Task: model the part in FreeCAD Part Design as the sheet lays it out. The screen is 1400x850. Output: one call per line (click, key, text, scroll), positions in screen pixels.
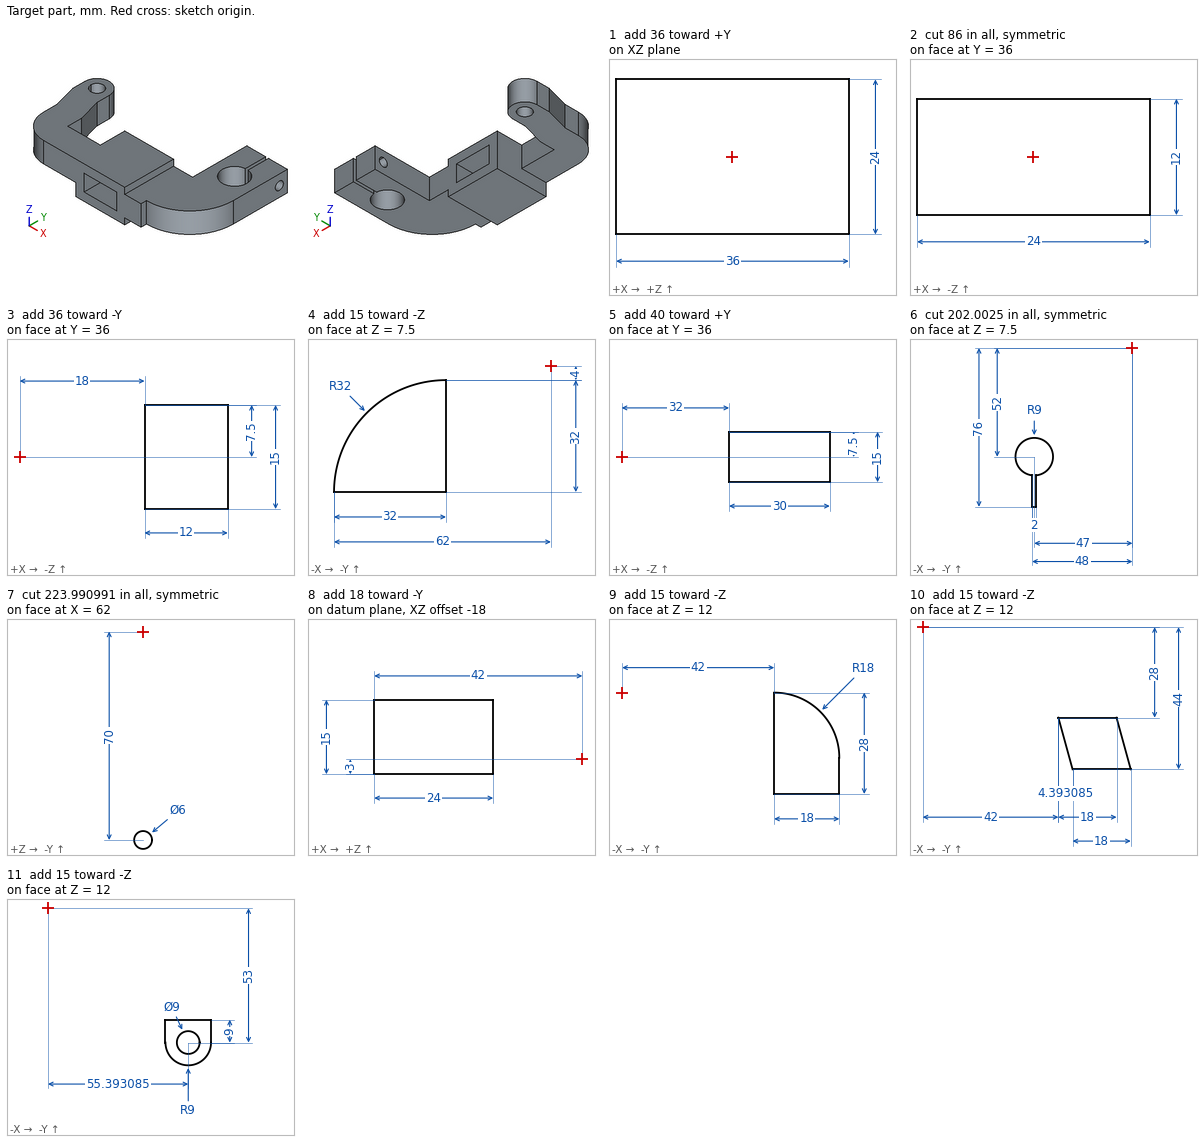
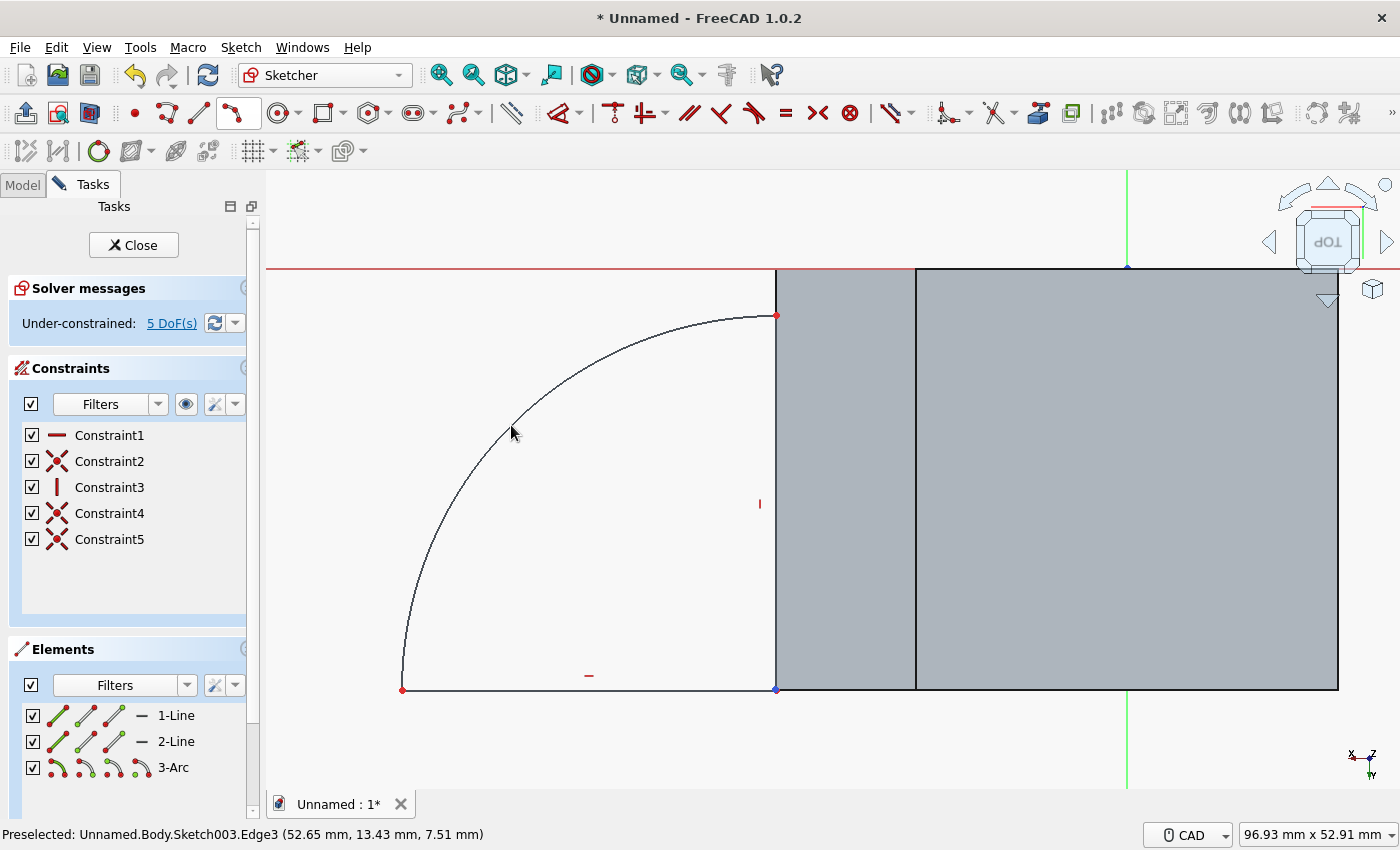
key(d)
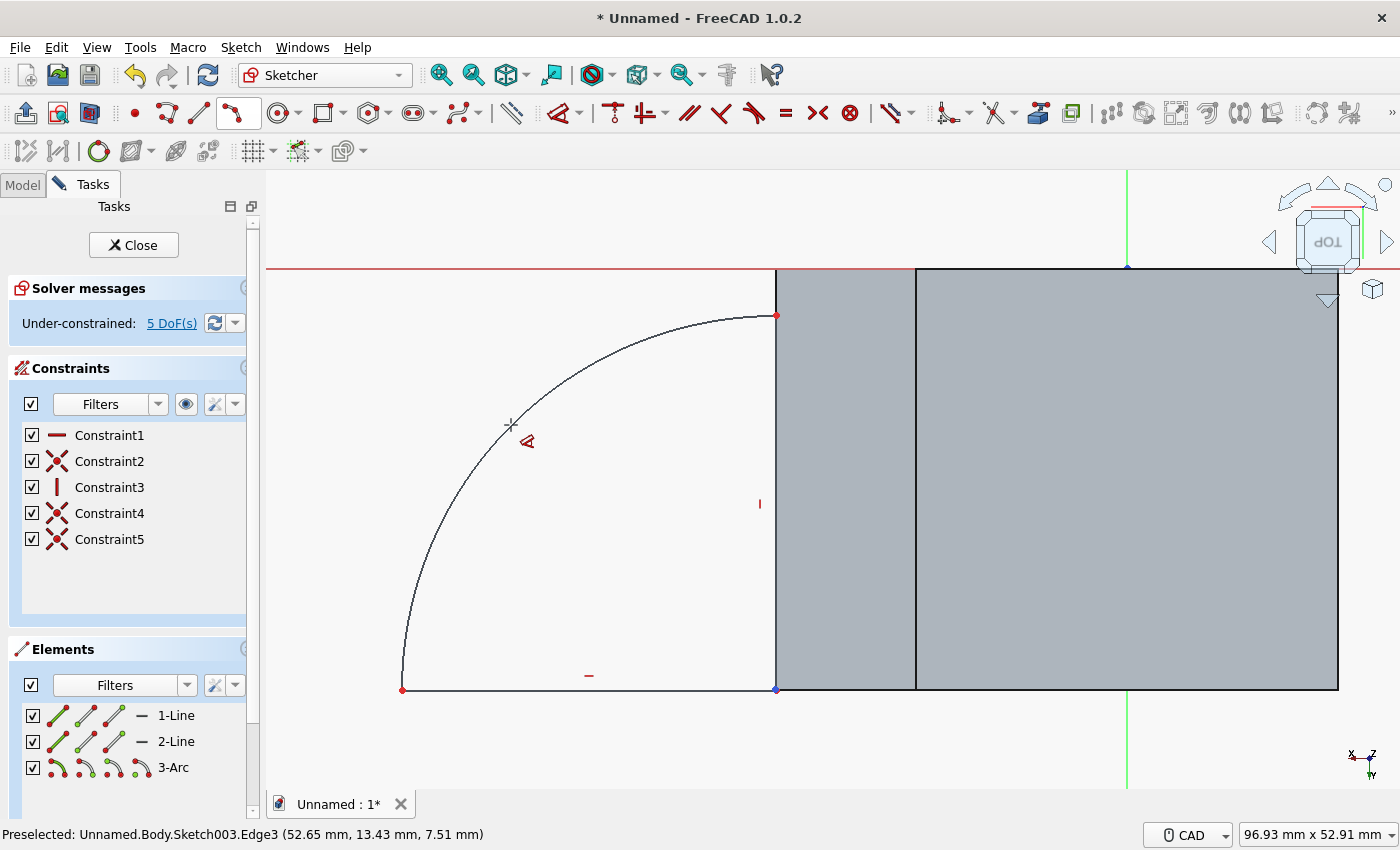
click(606, 357)
click(591, 328)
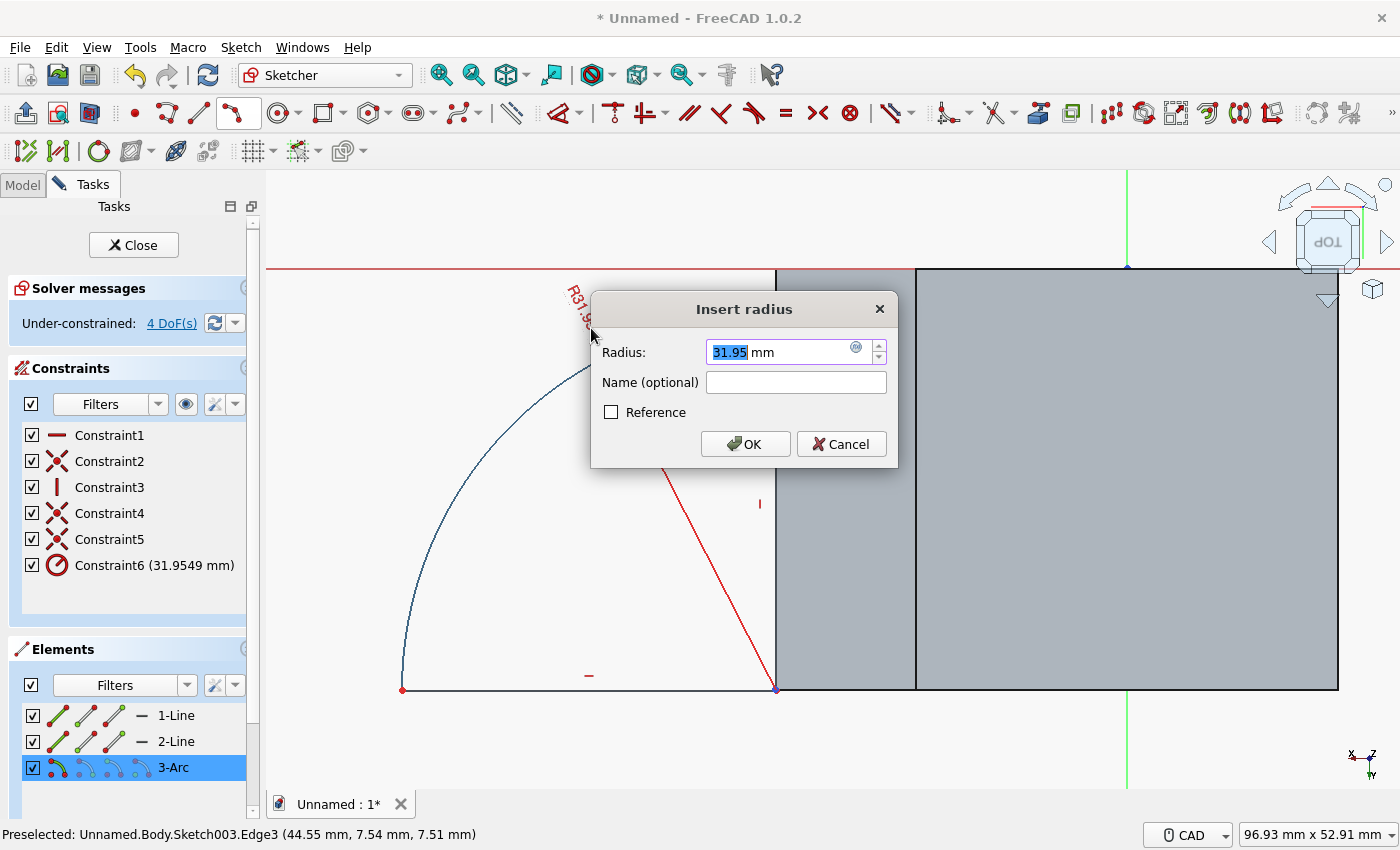
text(32)
key(Return)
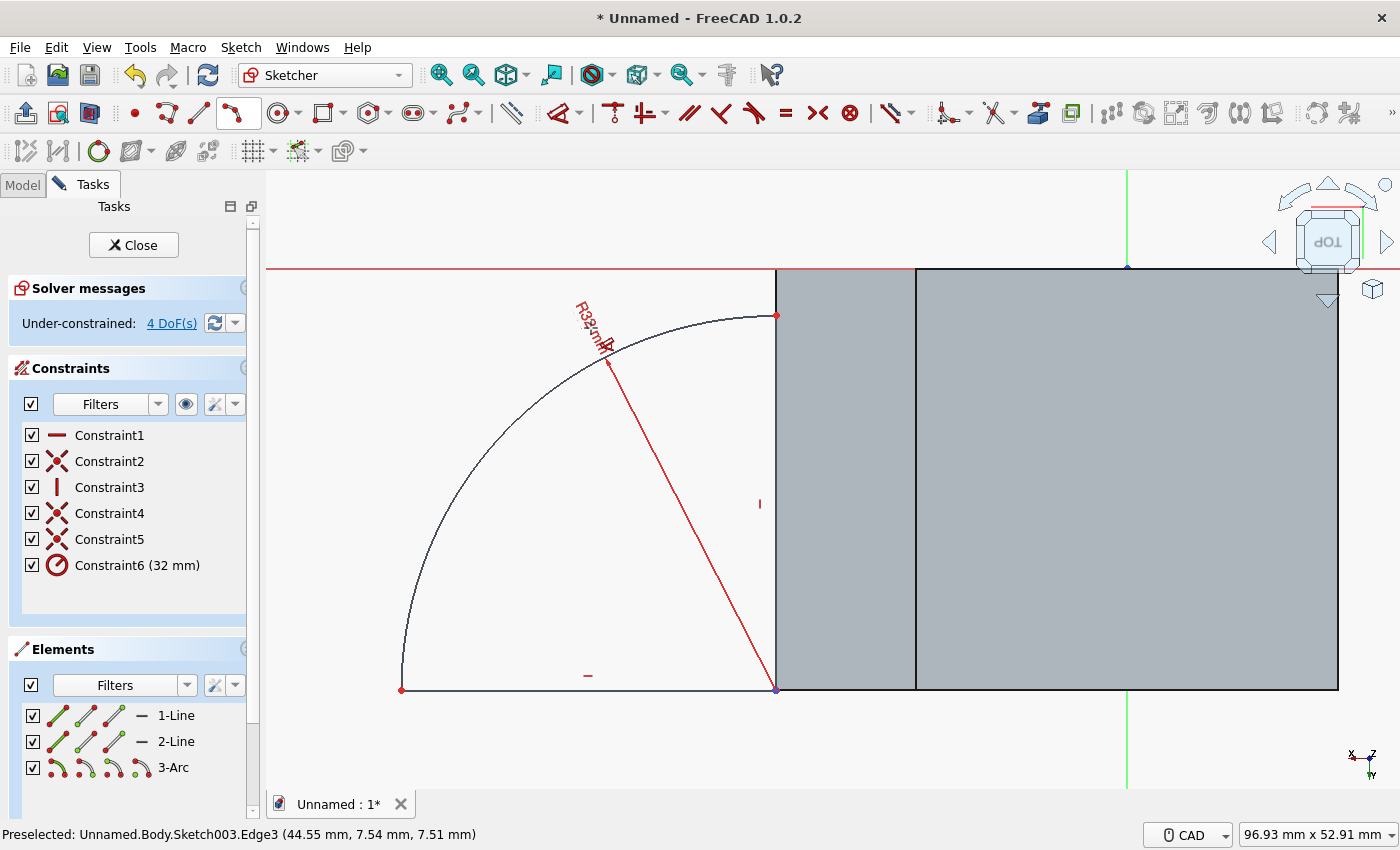
click(514, 691)
click(589, 725)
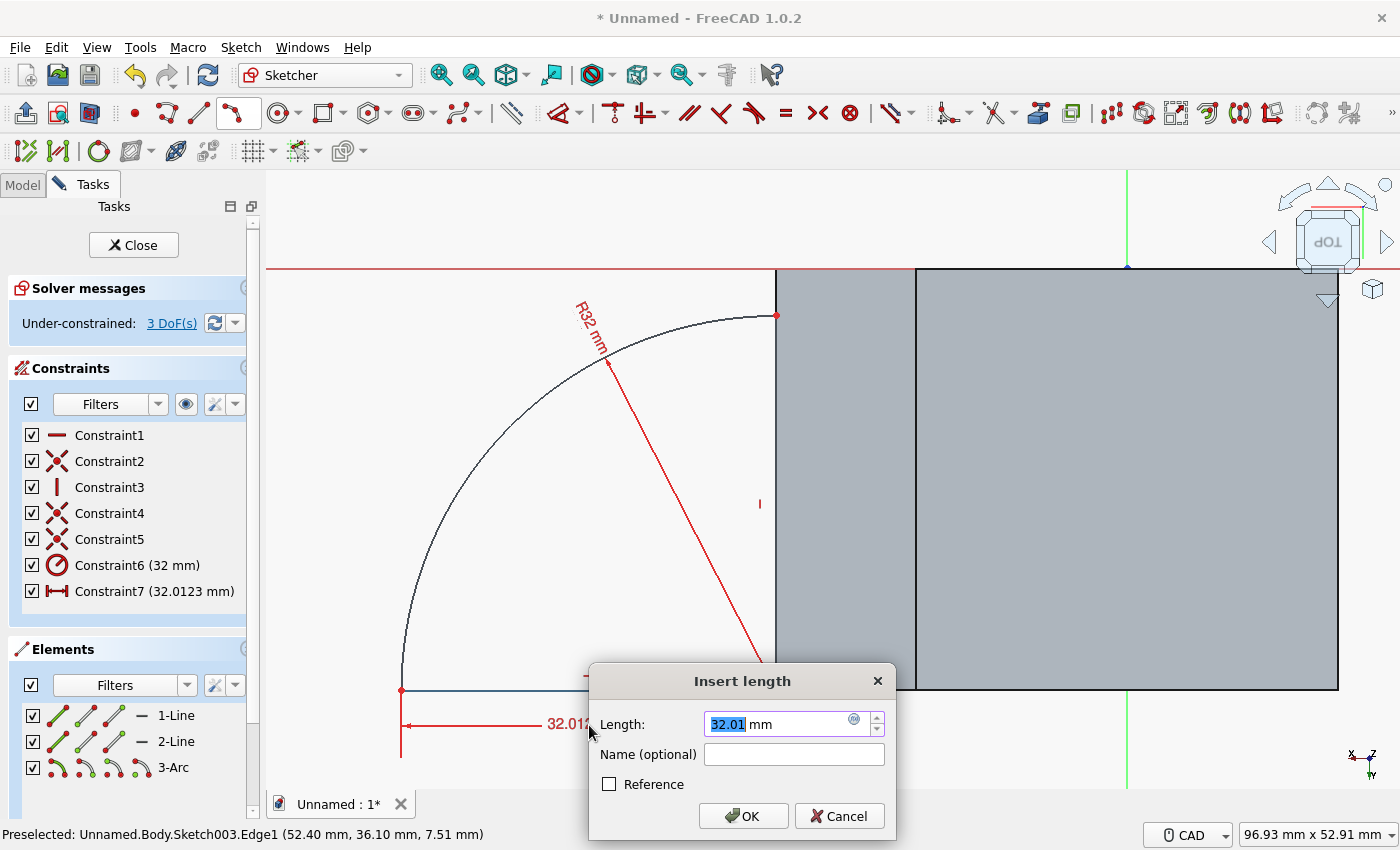
text(32)
key(Return)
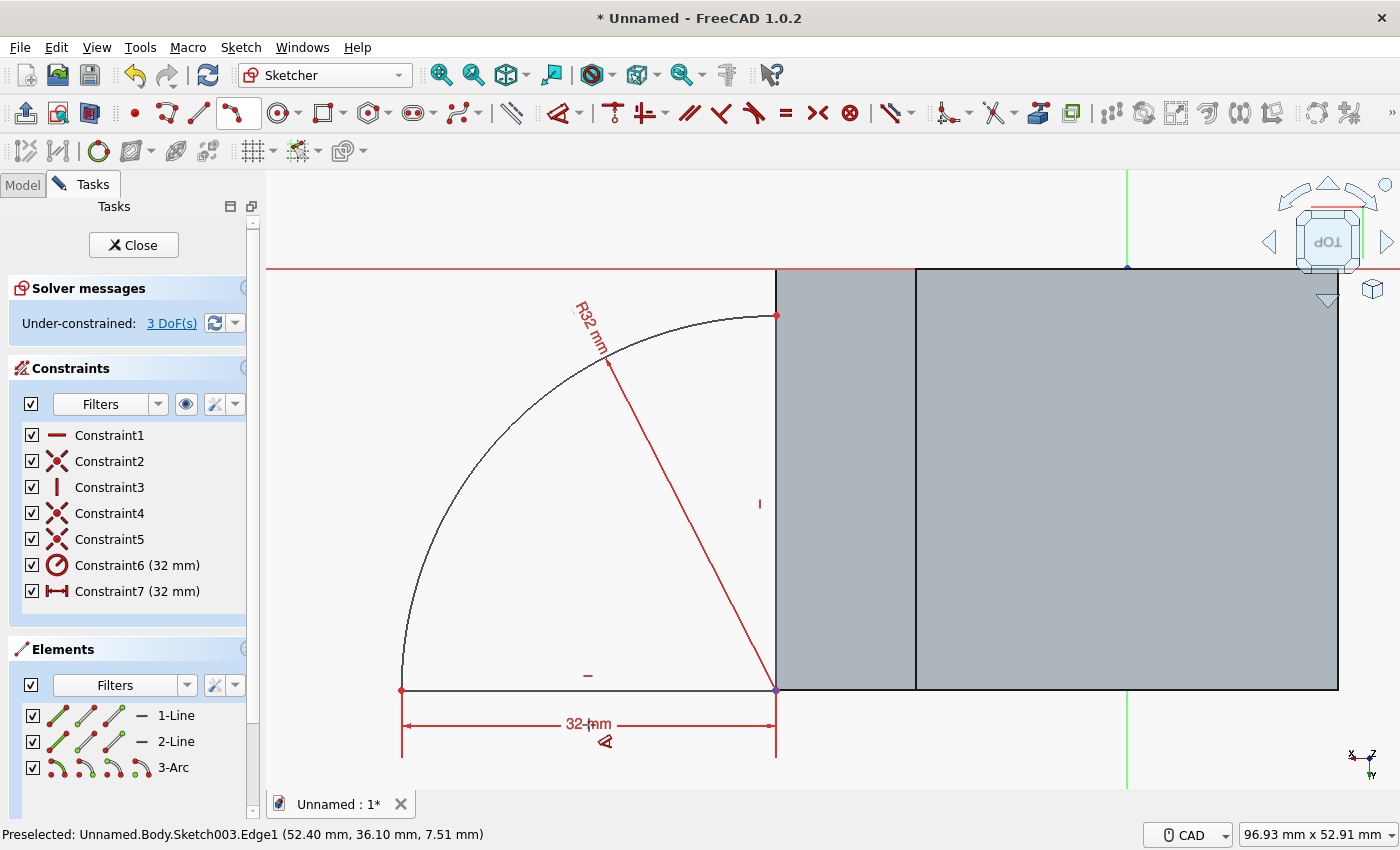
click(776, 578)
click(810, 503)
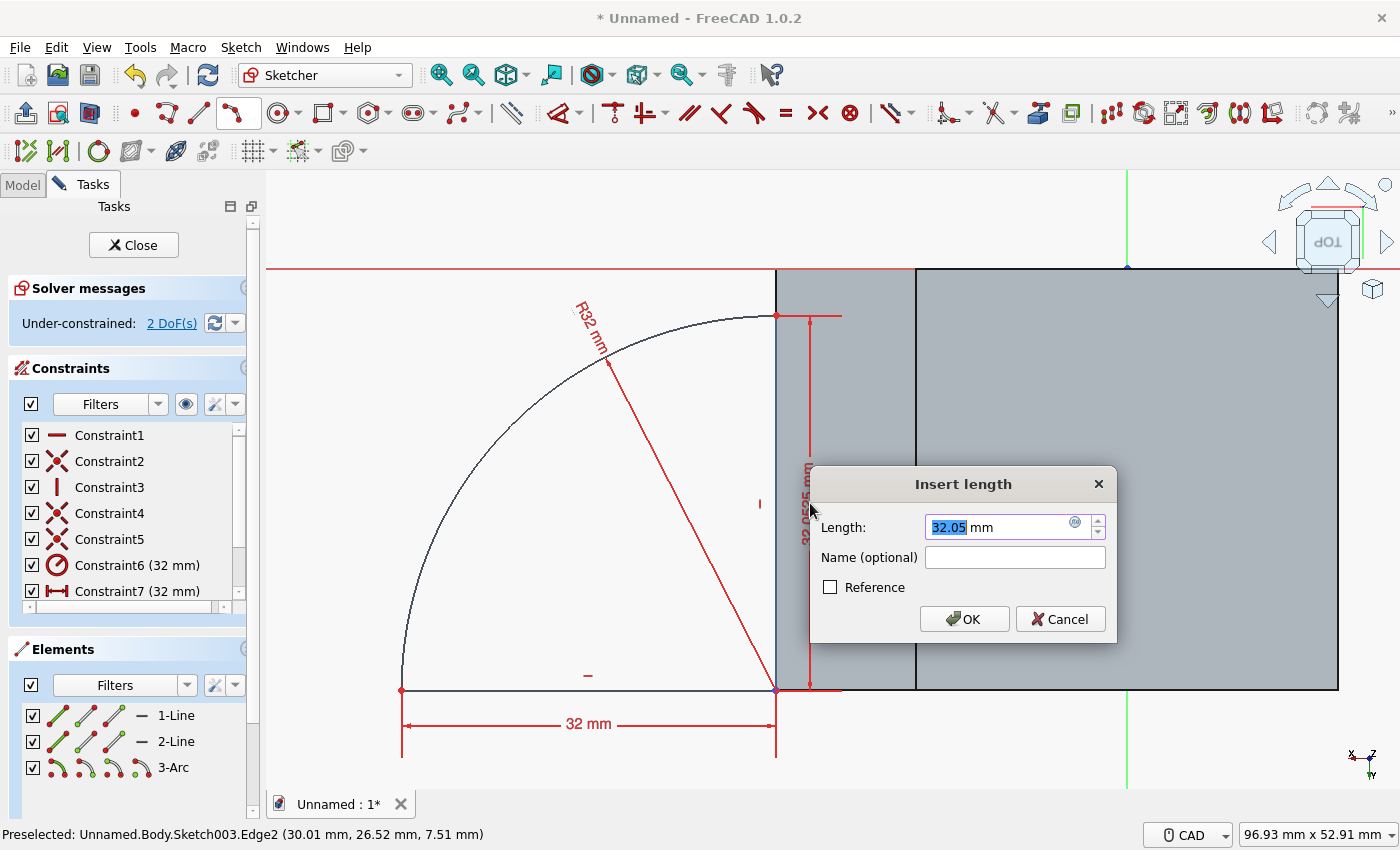
text(32)
key(Return)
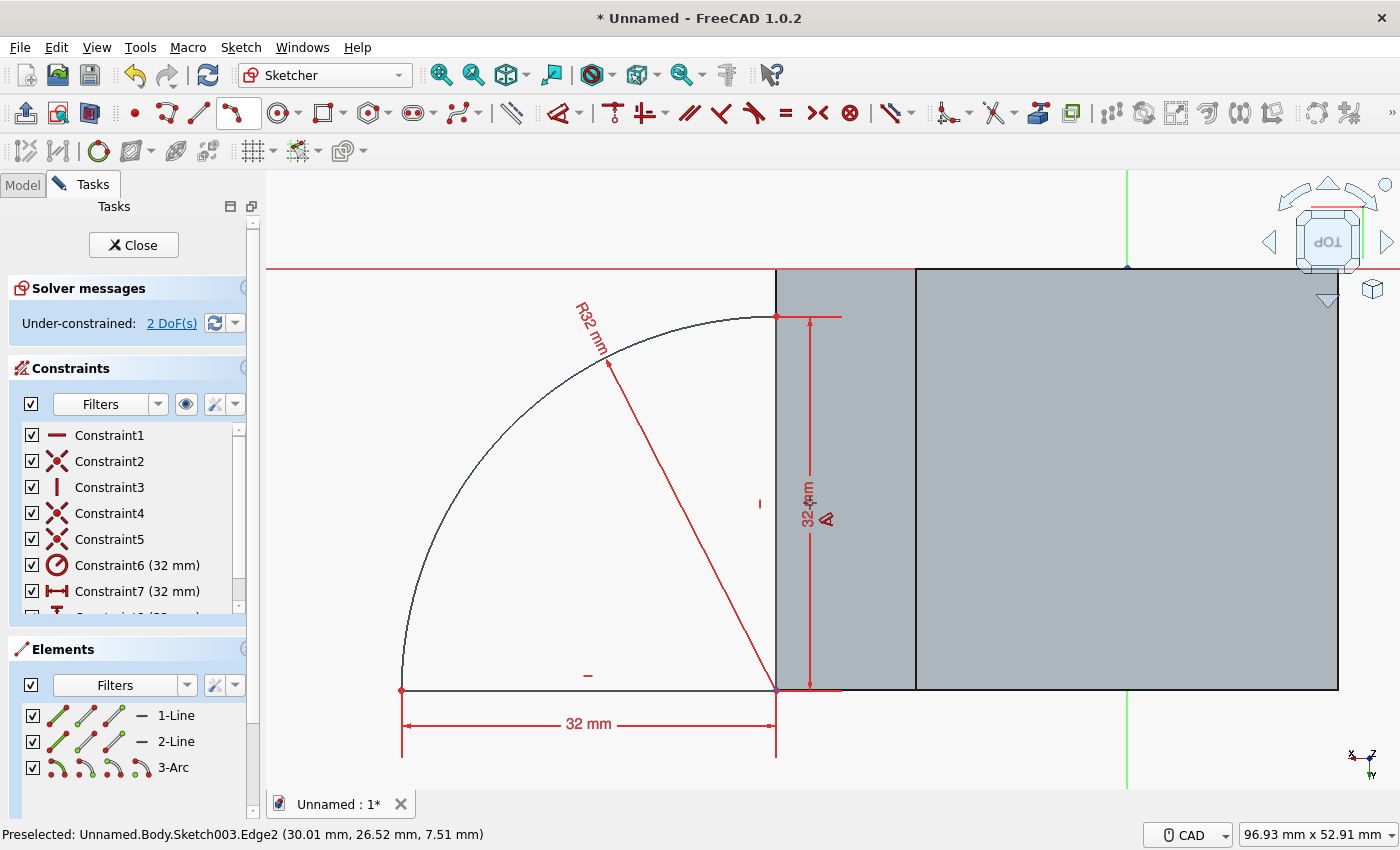
click(776, 317)
click(1161, 293)